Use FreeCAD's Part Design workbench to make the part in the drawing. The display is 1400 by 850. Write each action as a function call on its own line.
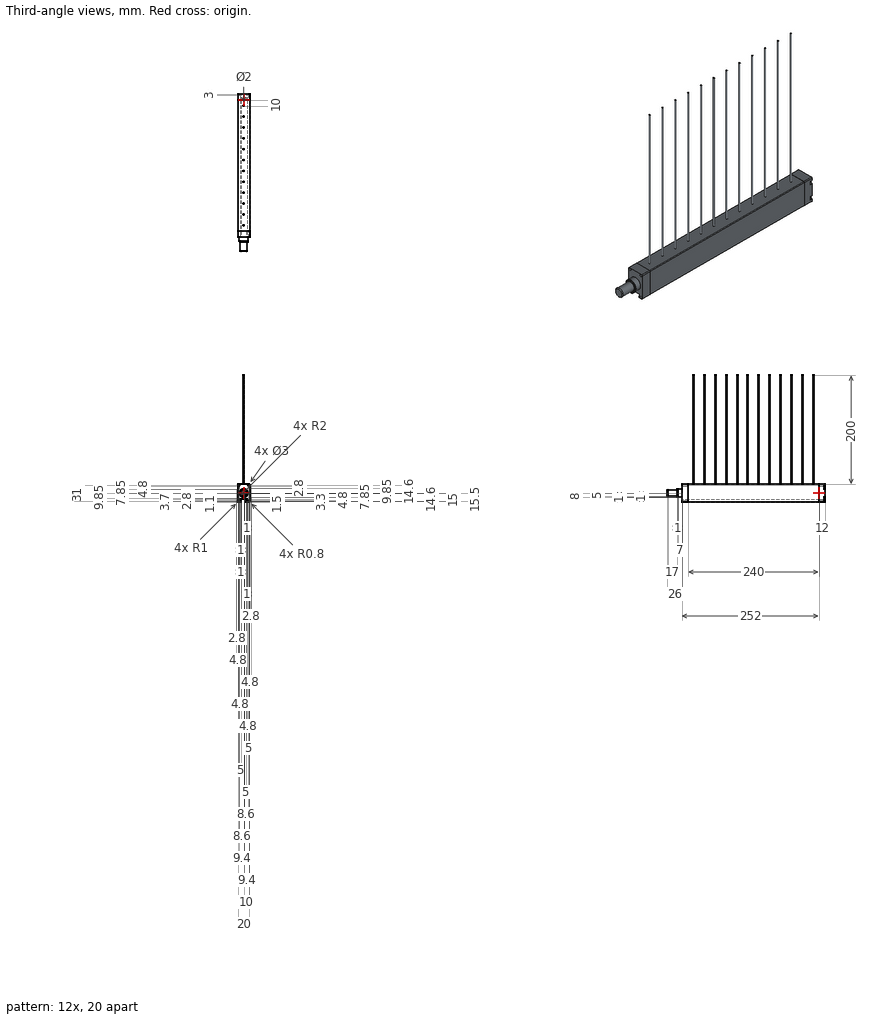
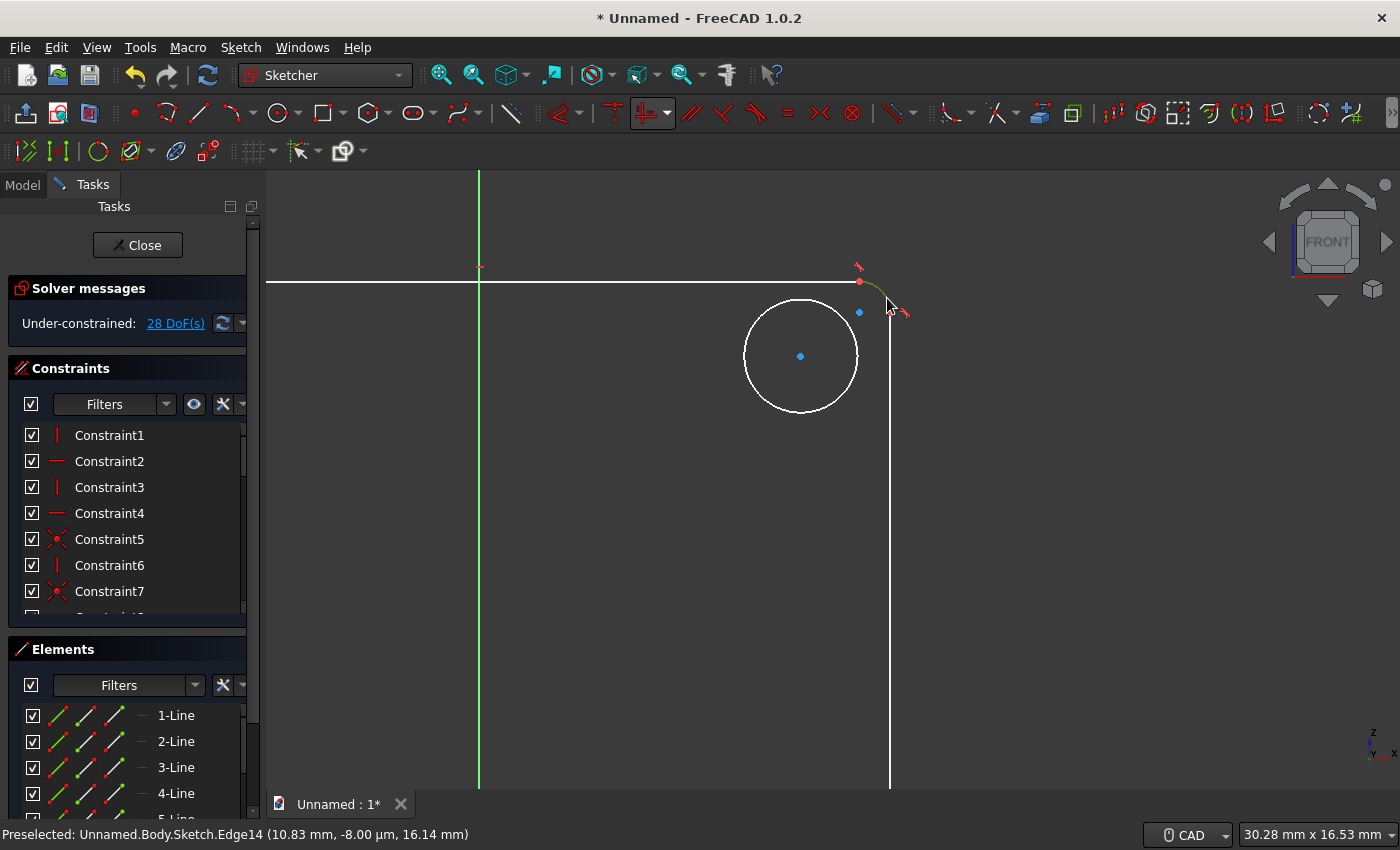
scroll(887, 298, down, 6)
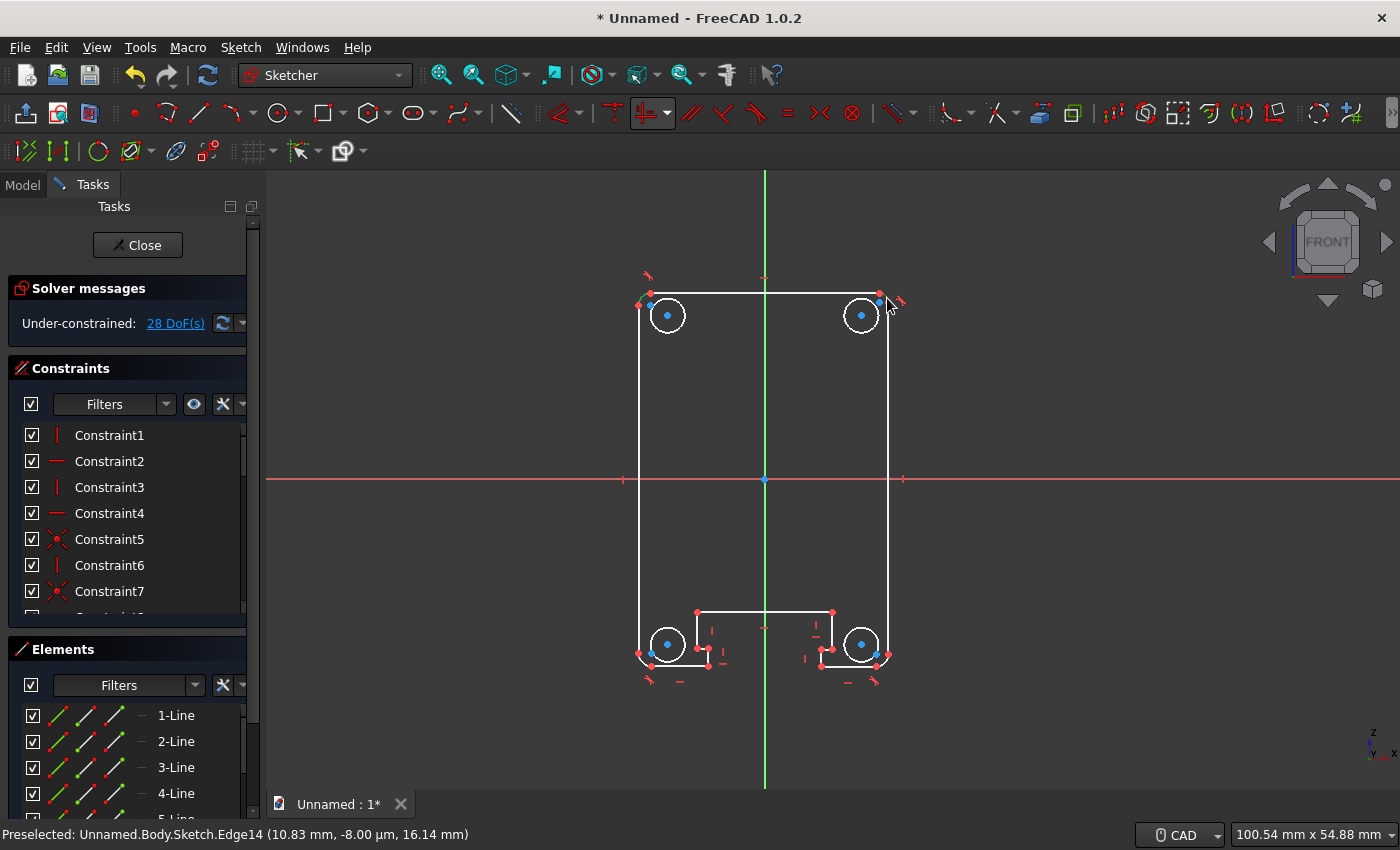
scroll(882, 665, up, 5)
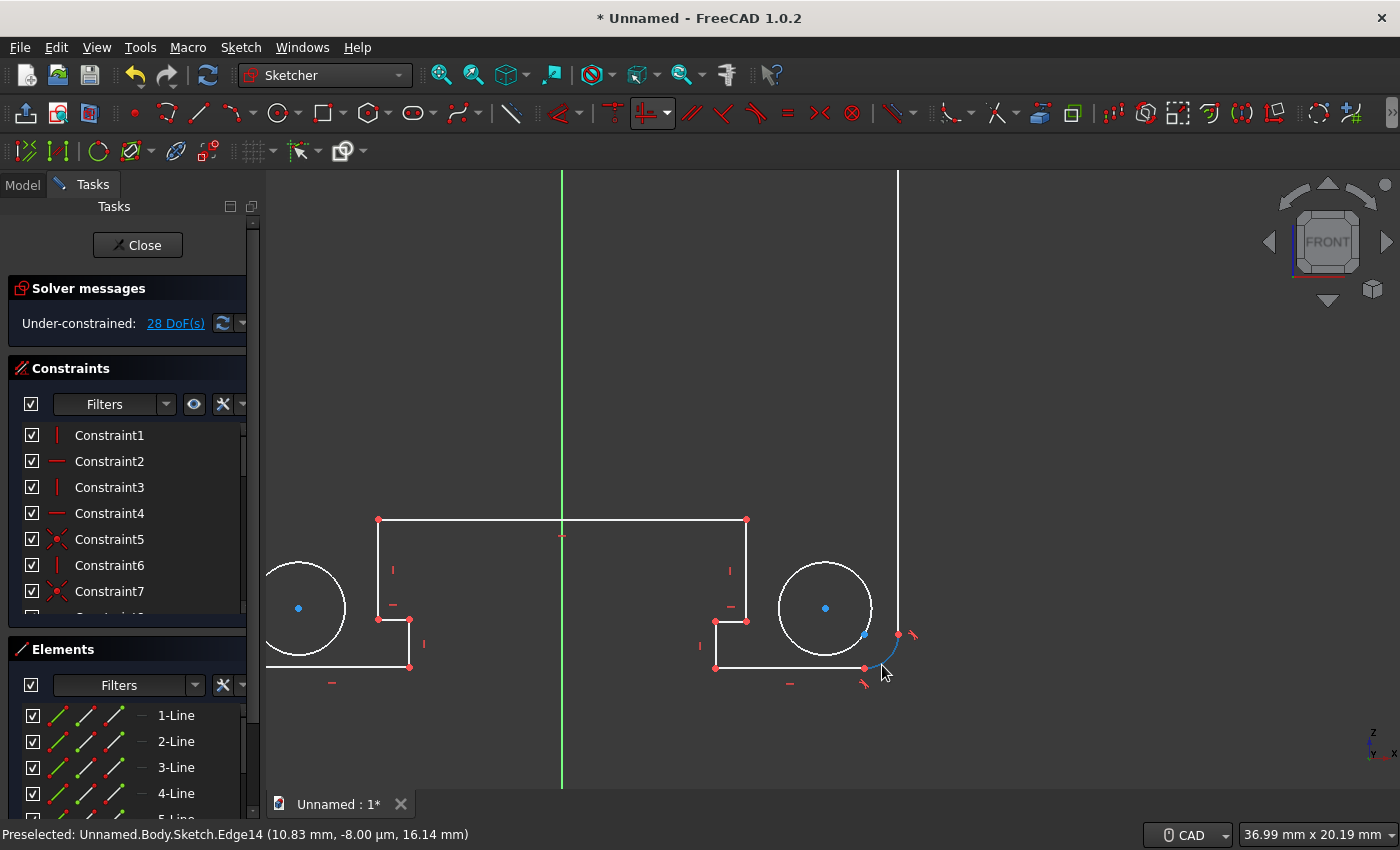
click(880, 665)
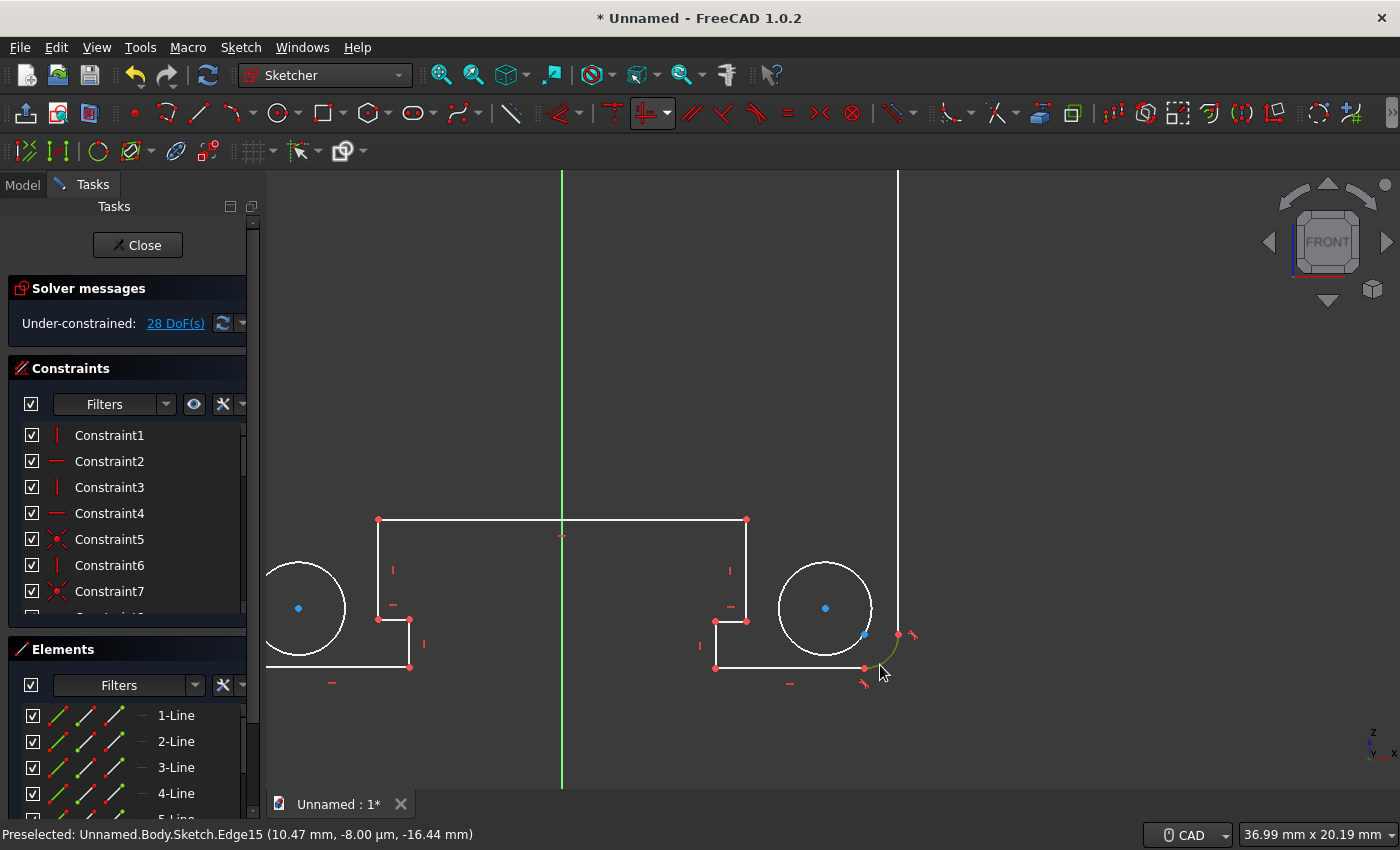
scroll(882, 666, down, 5)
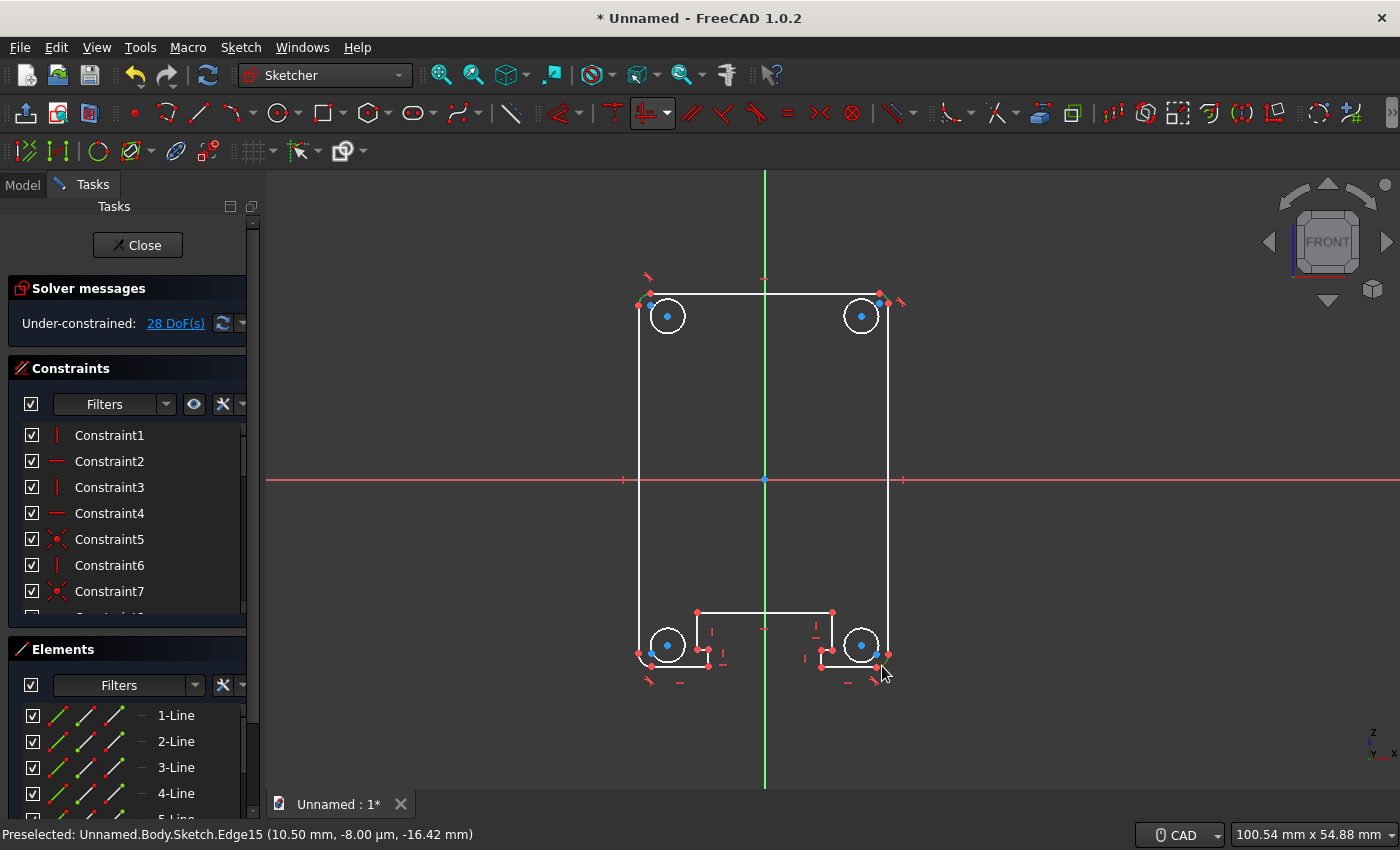
scroll(640, 660, up, 5)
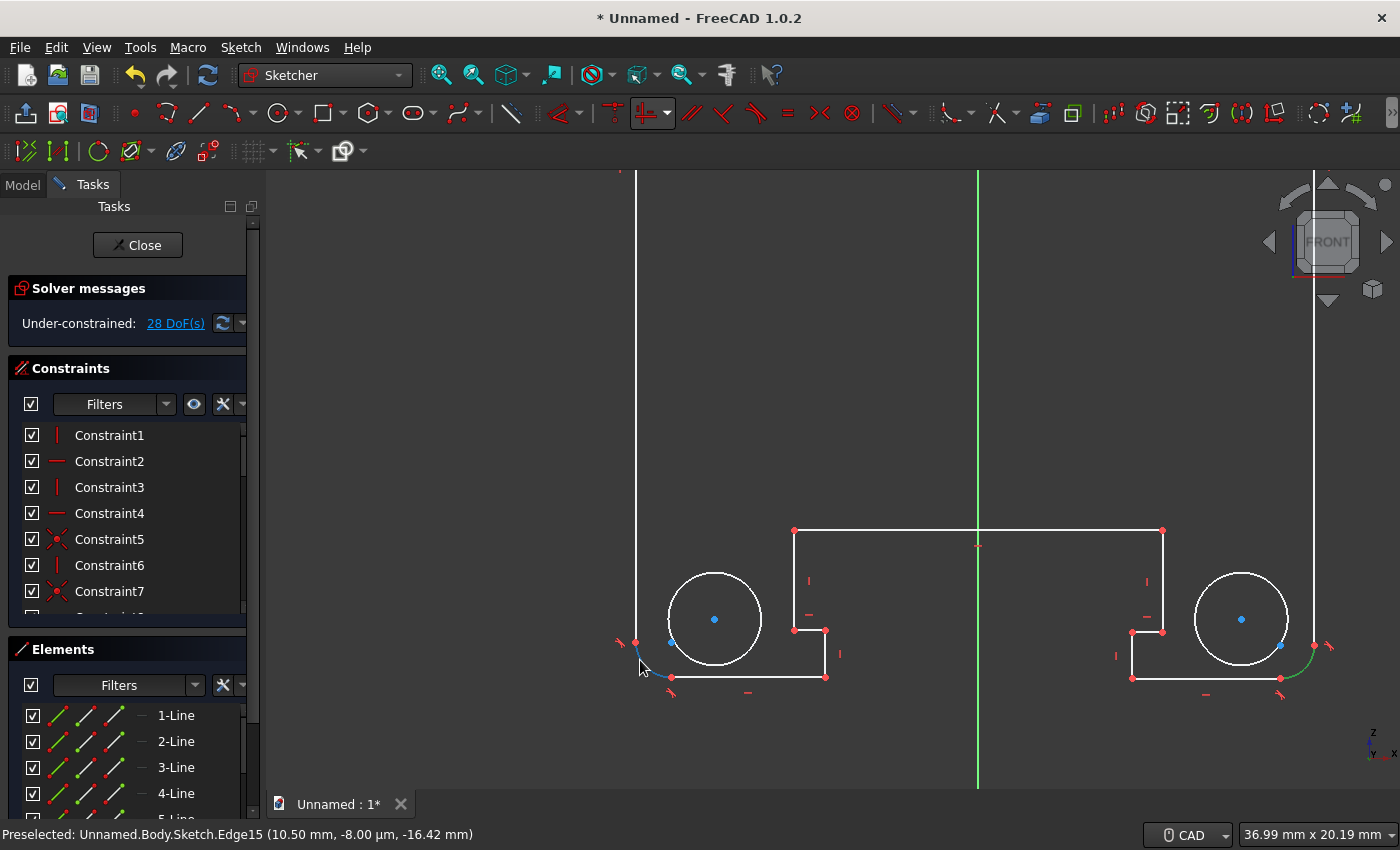
click(640, 658)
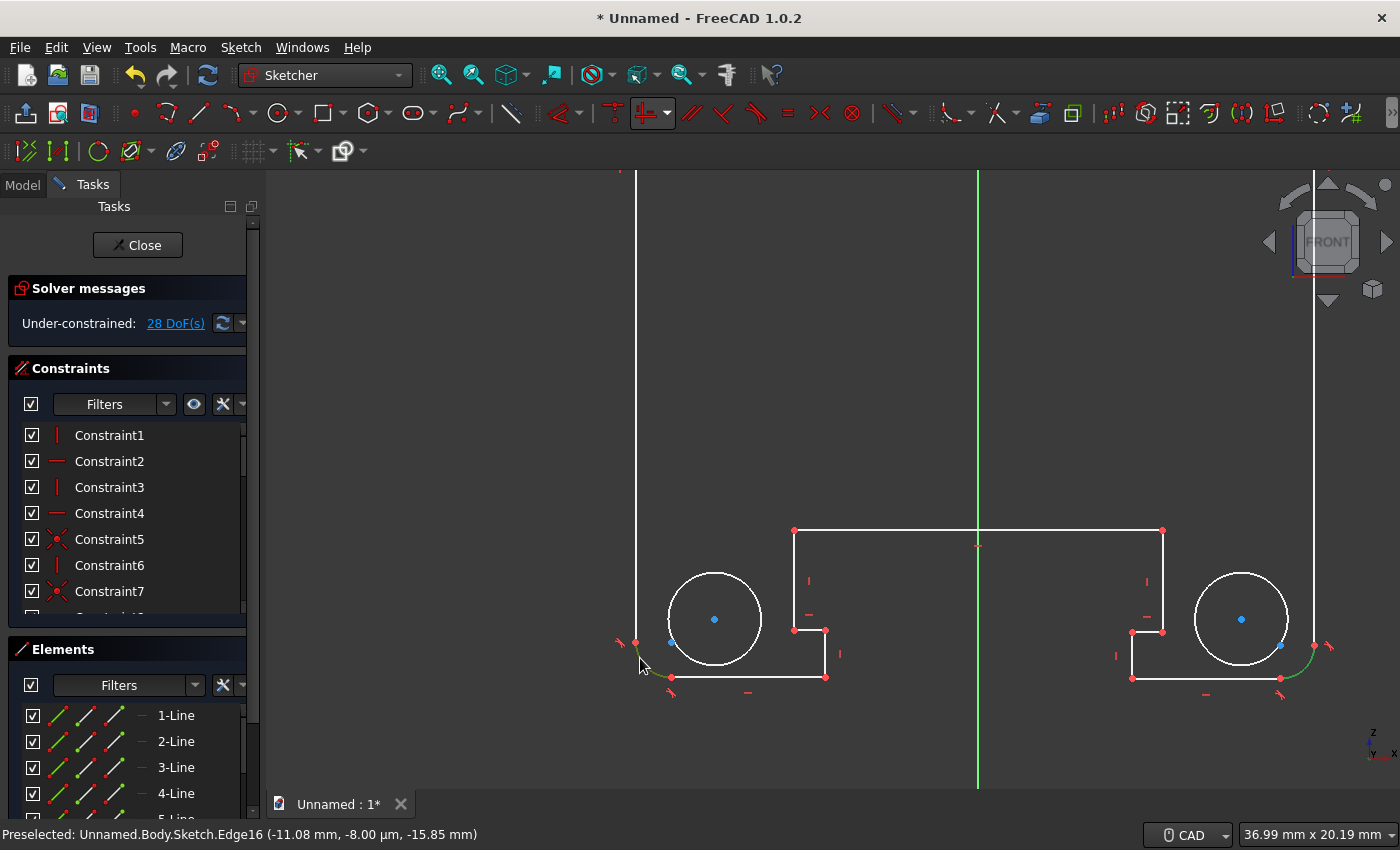
click(788, 114)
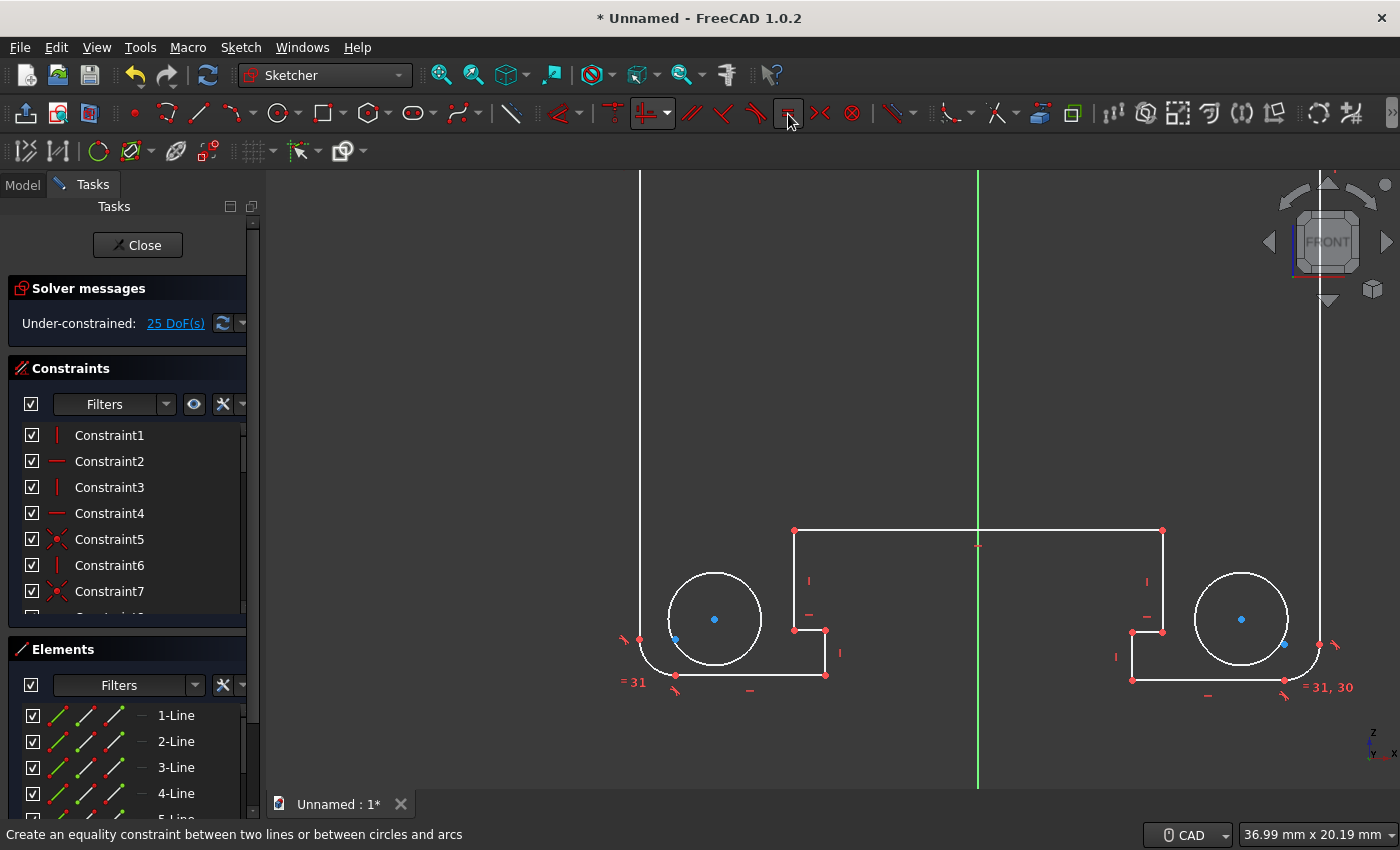
scroll(640, 660, down, 5)